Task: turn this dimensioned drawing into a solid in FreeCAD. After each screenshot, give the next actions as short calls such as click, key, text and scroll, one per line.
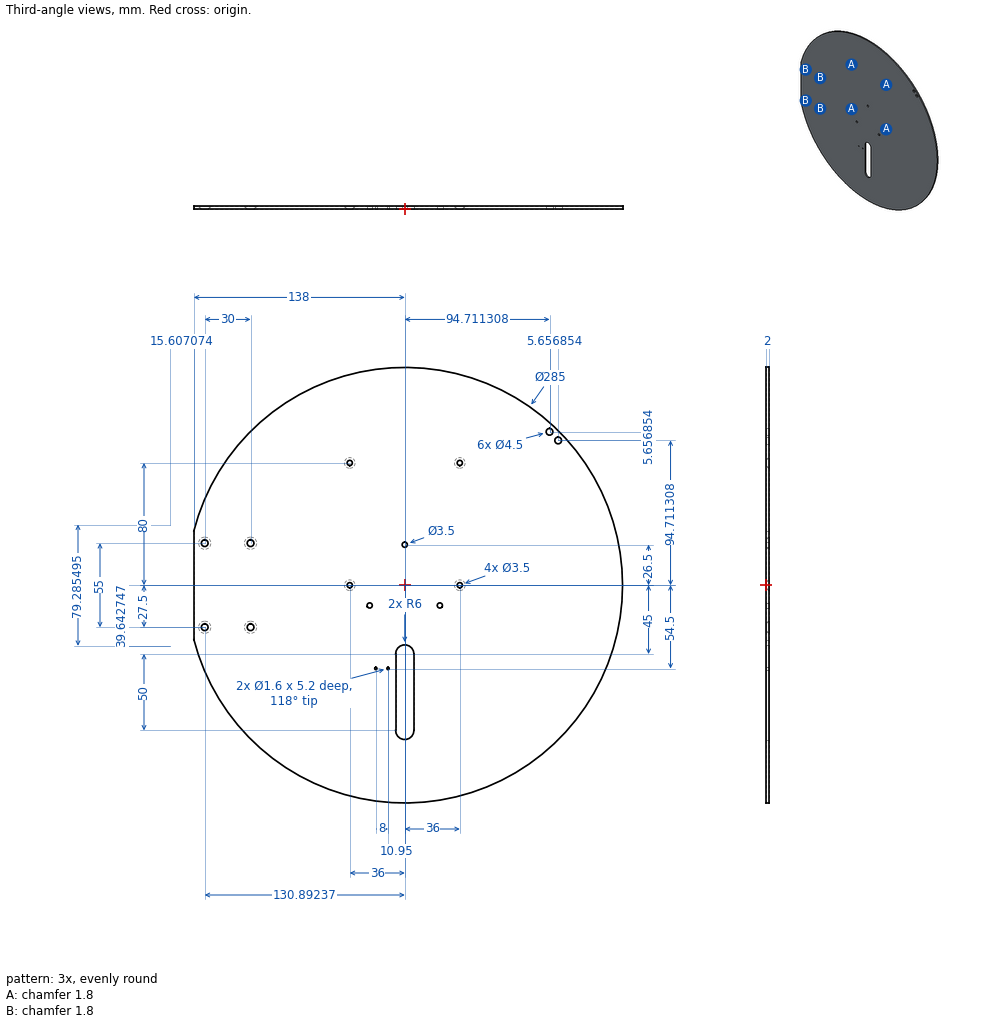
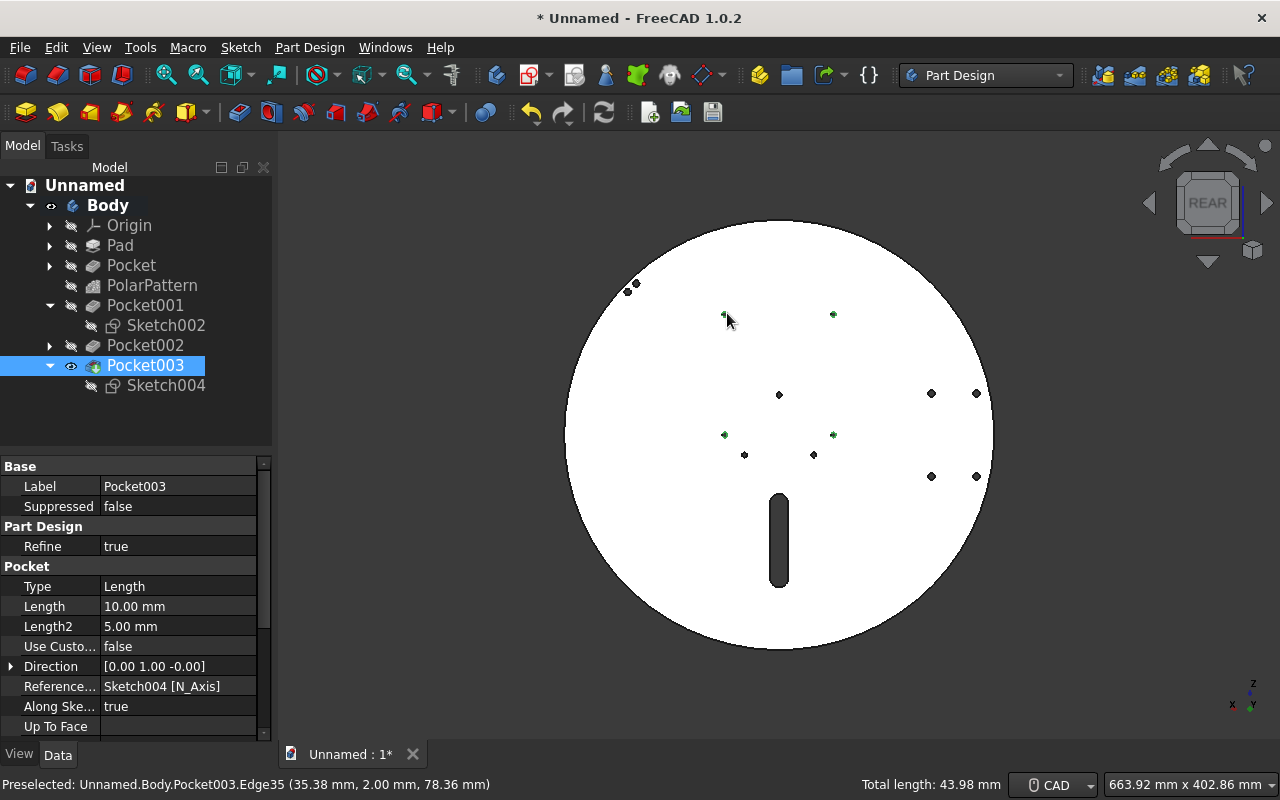
click(58, 76)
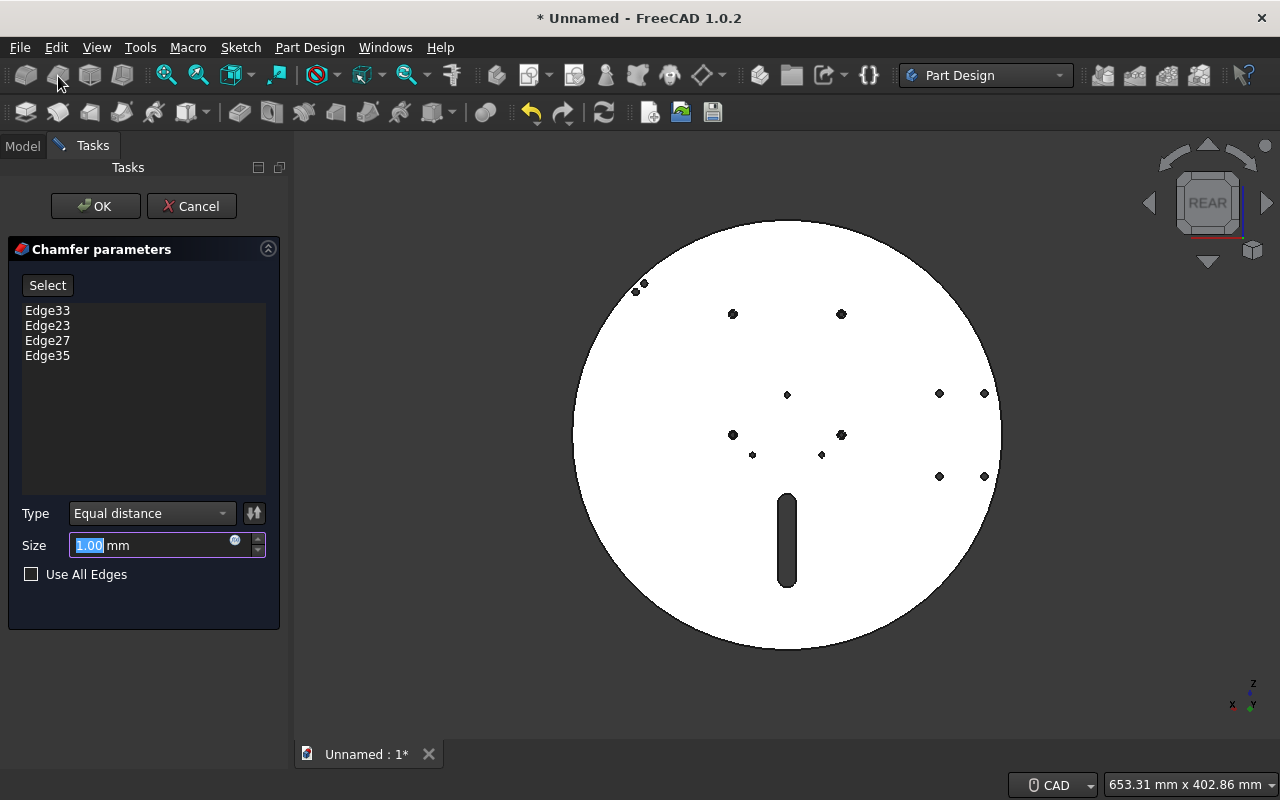
text(1.8)
key(Tab)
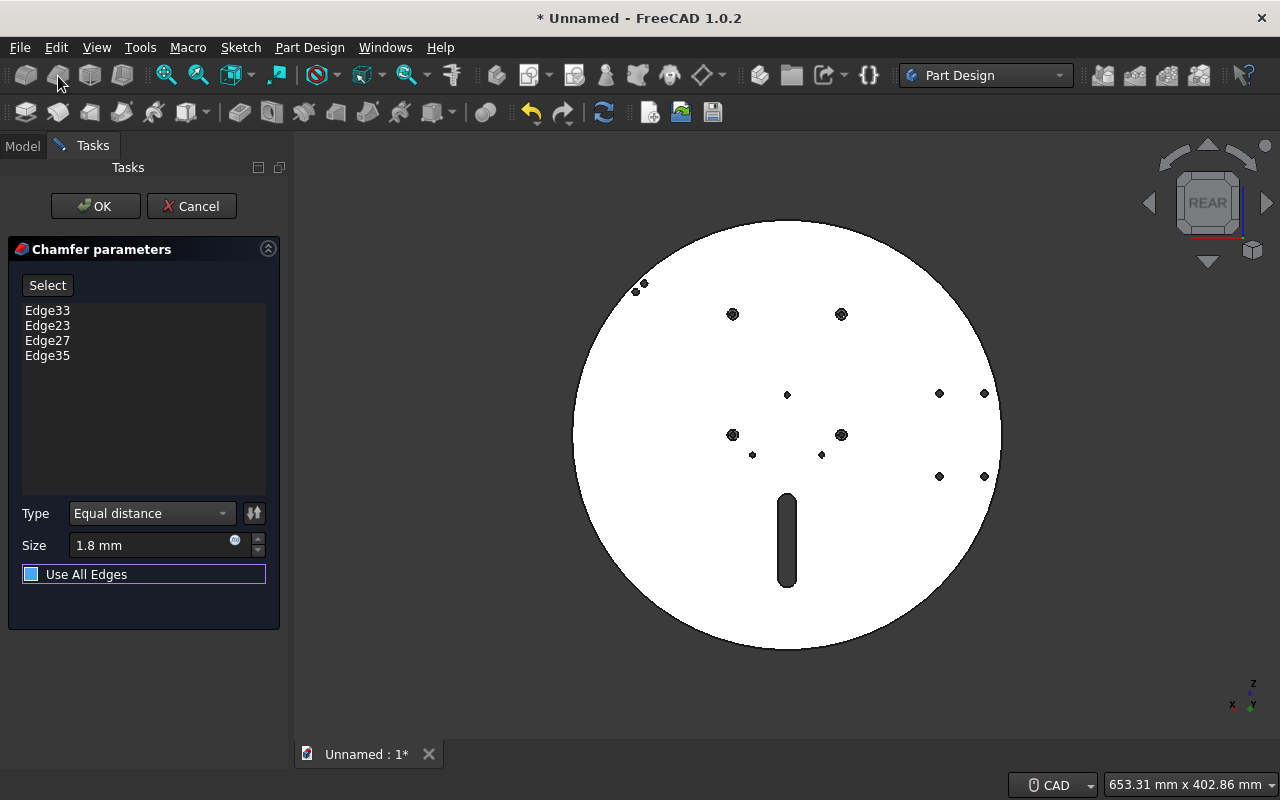
click(96, 206)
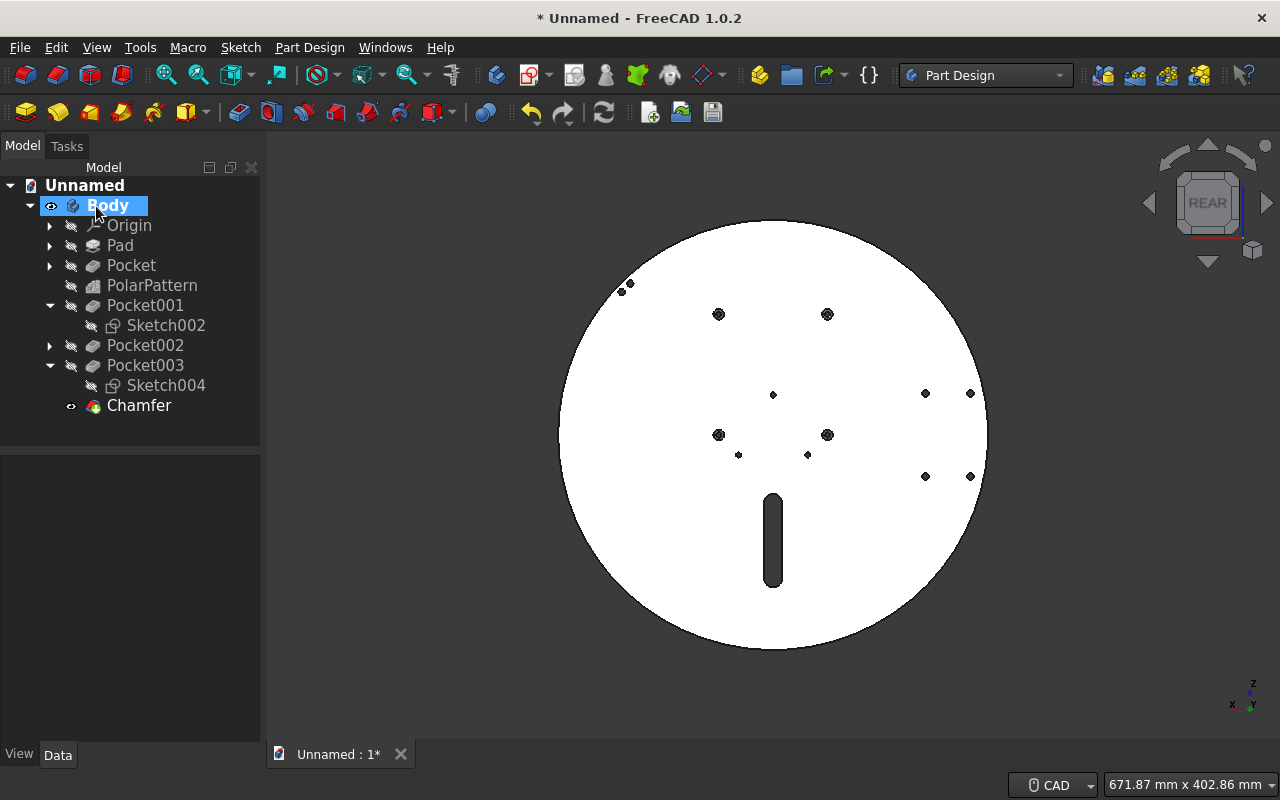
click(974, 476)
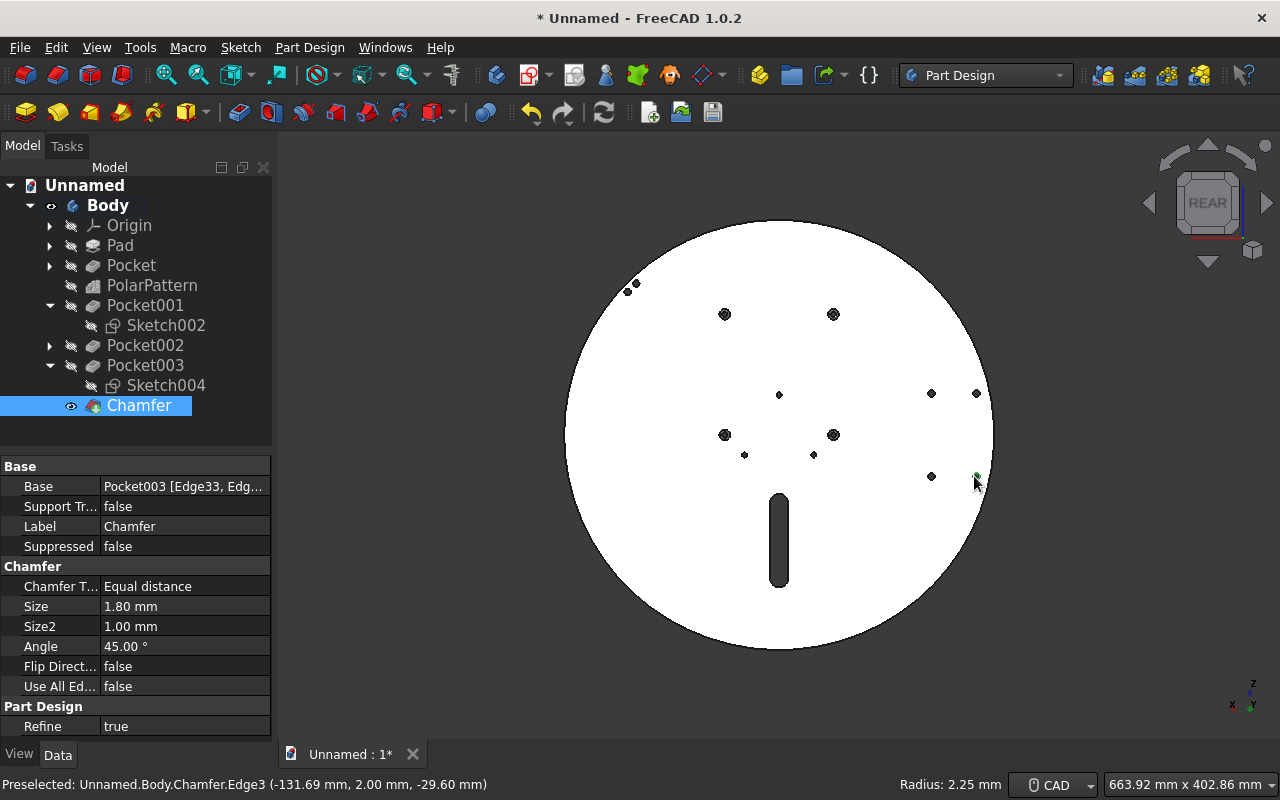
click(980, 392, ctrl)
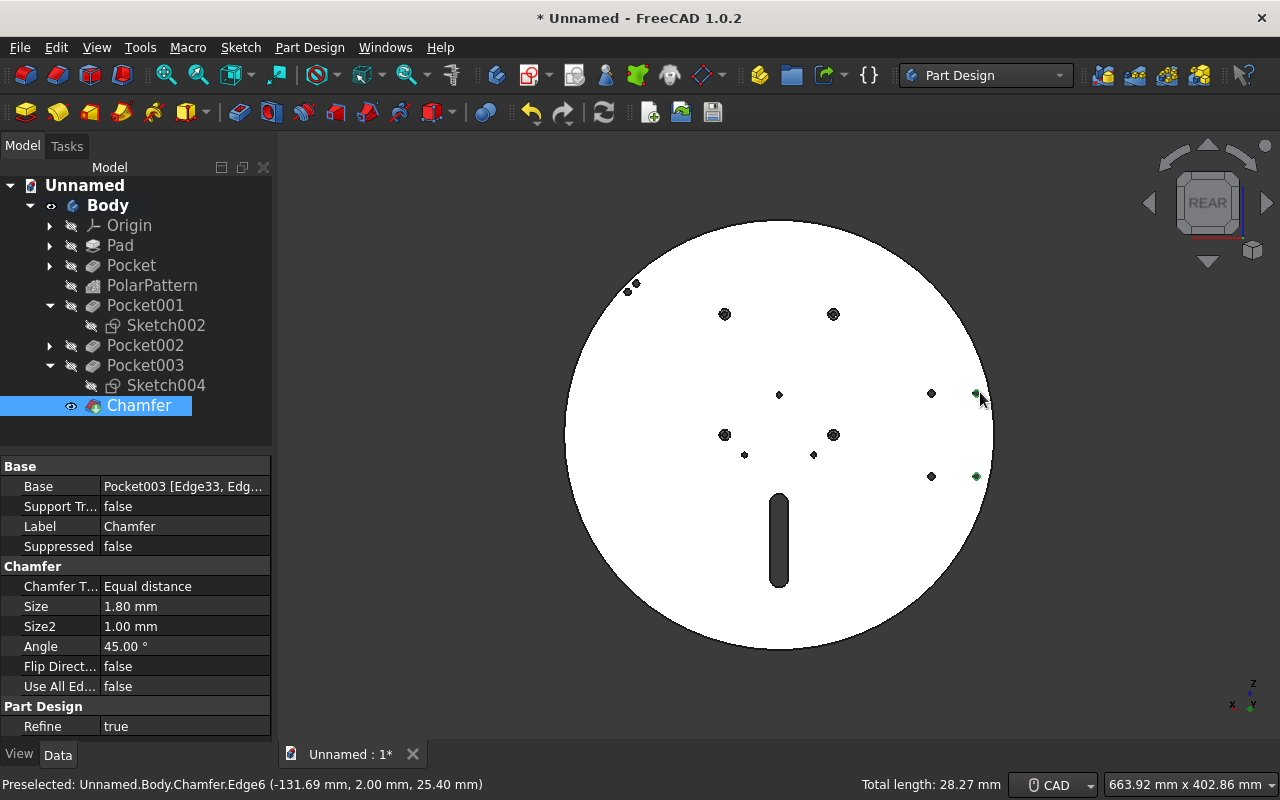
click(935, 392, ctrl)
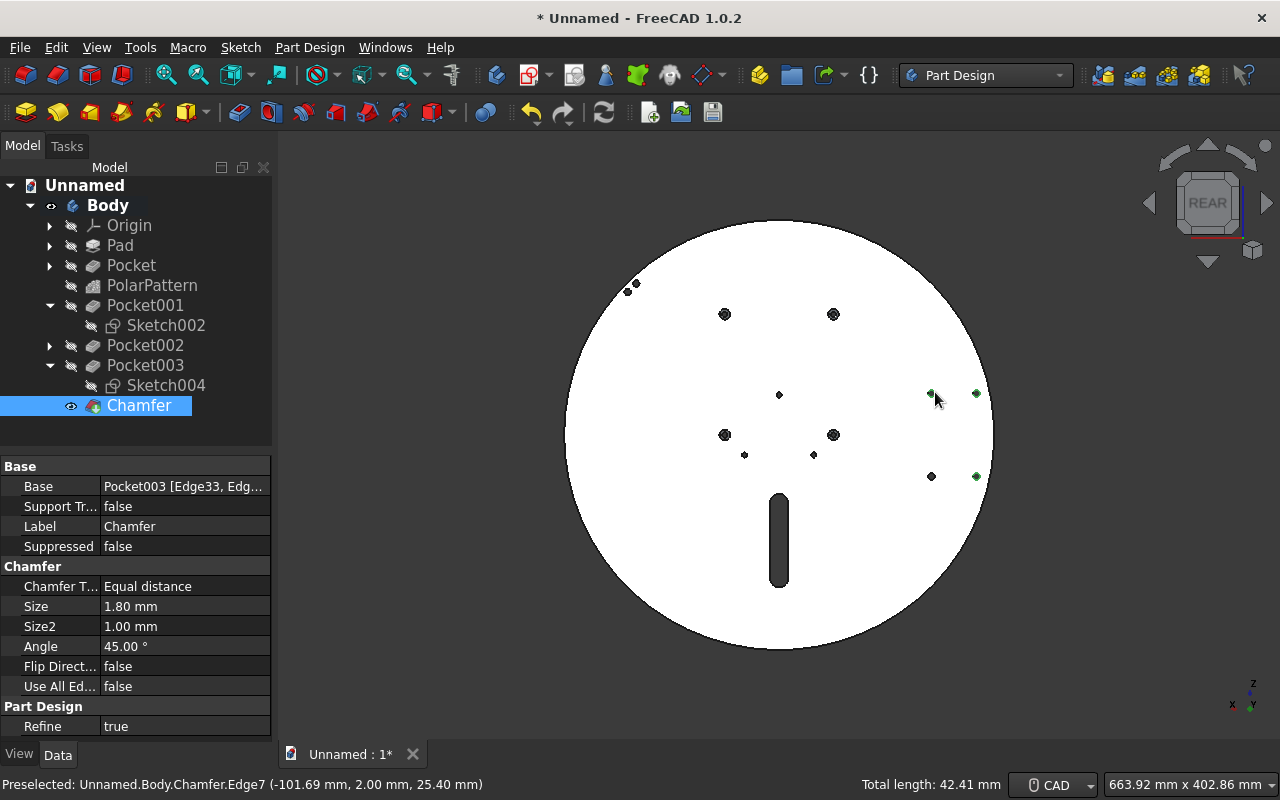
click(934, 474, ctrl)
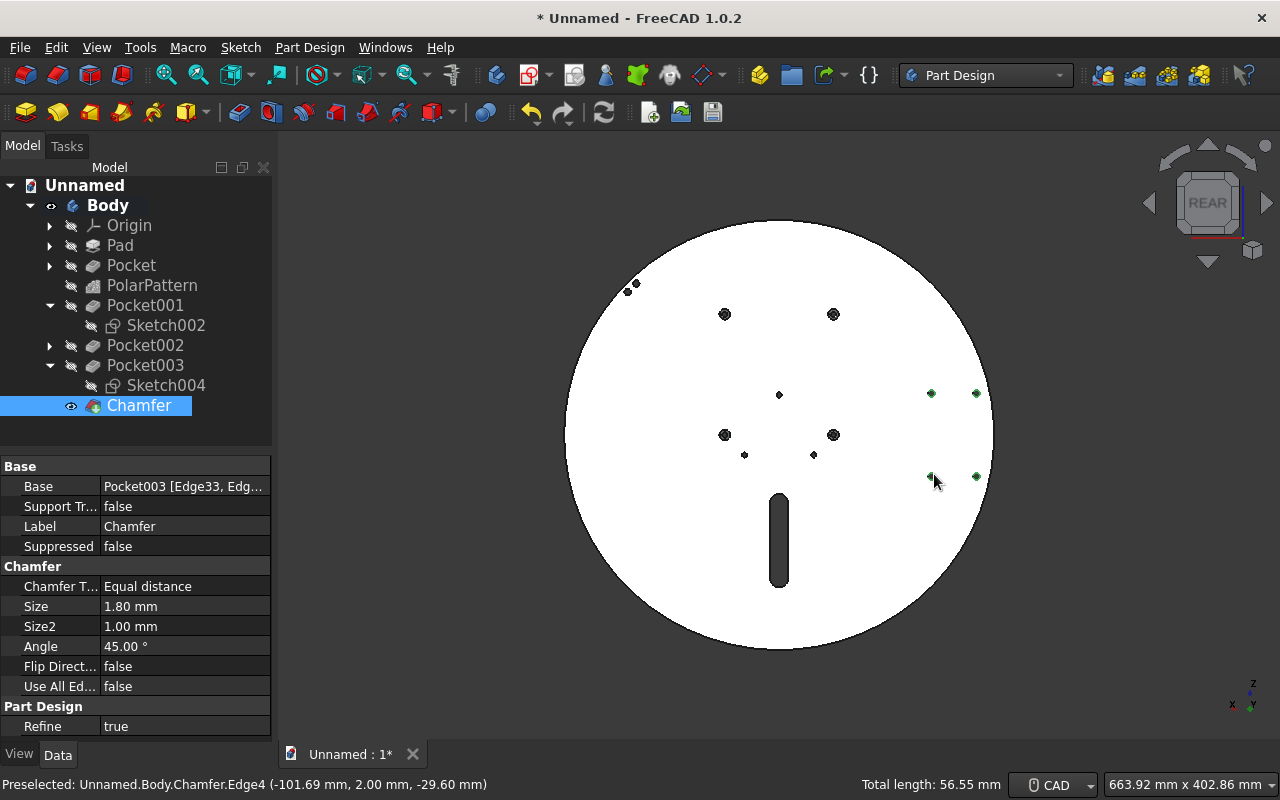
click(58, 76)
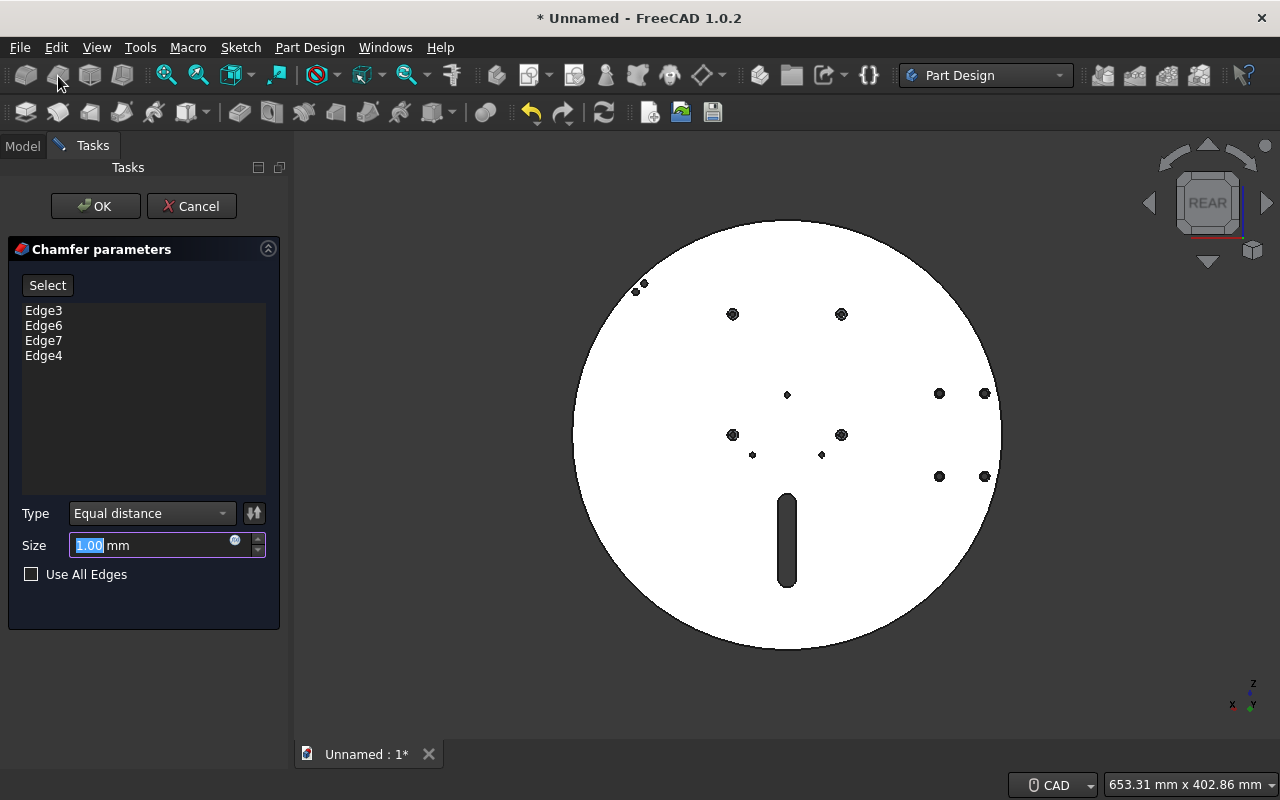
text(1.8)
key(Tab)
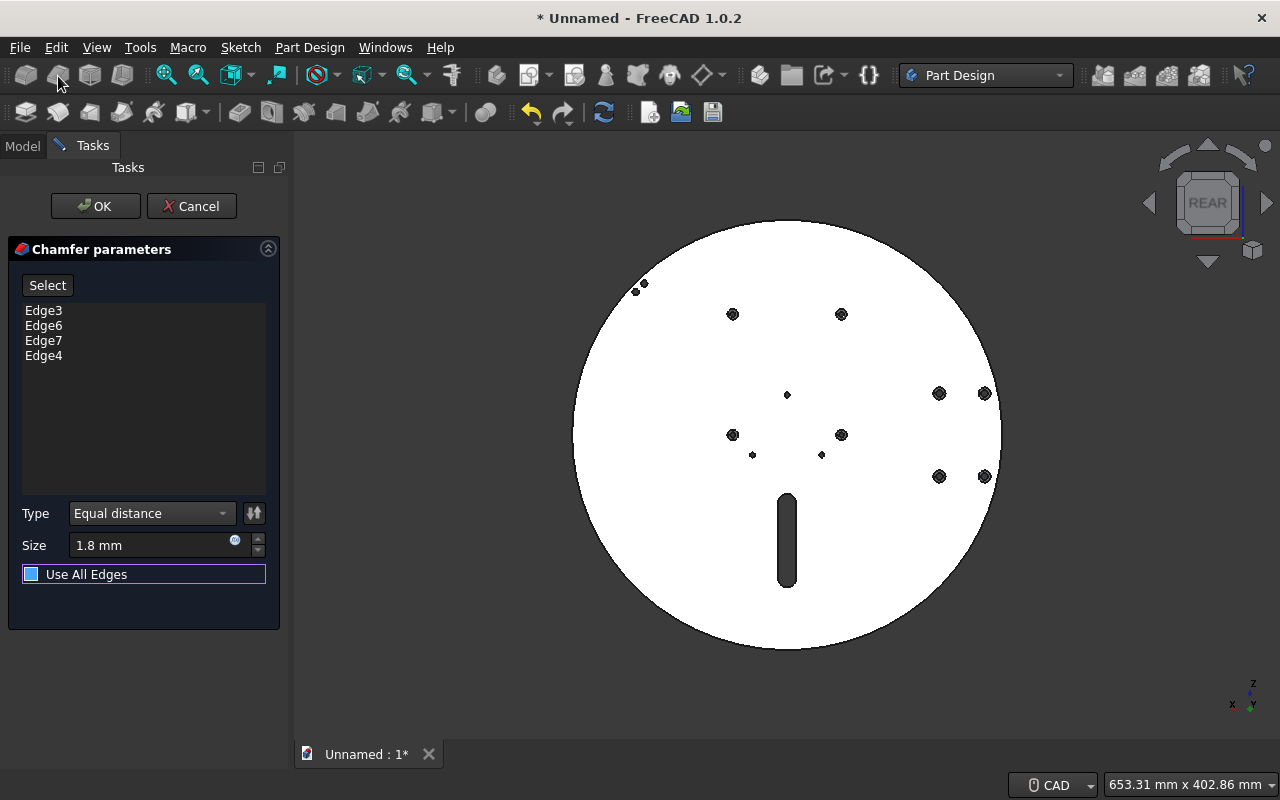
click(96, 206)